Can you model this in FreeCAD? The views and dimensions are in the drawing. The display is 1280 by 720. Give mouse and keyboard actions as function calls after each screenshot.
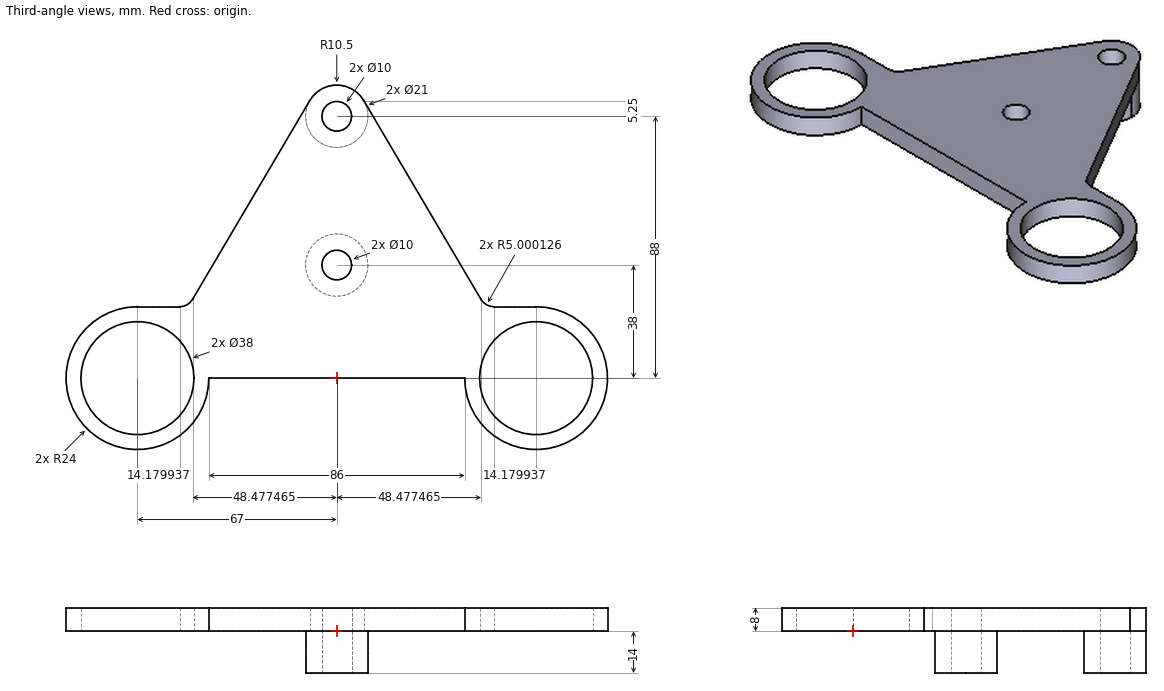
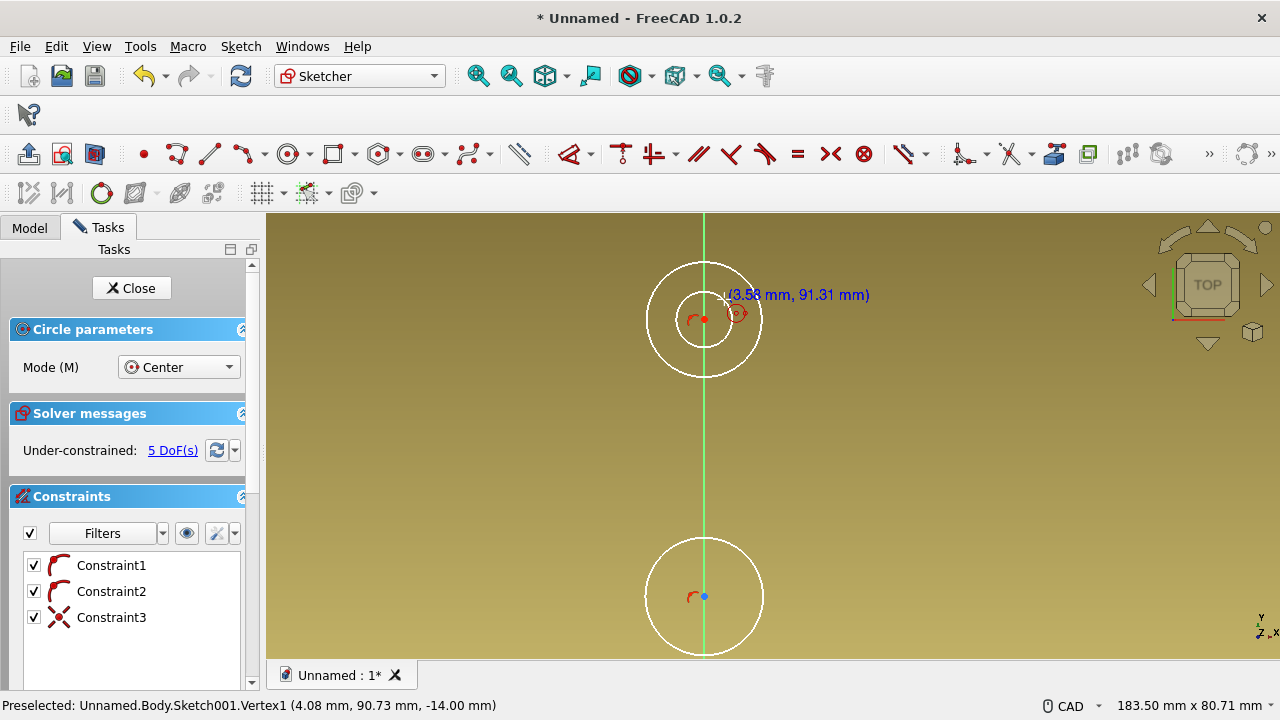
click(704, 597)
click(724, 575)
key(Escape)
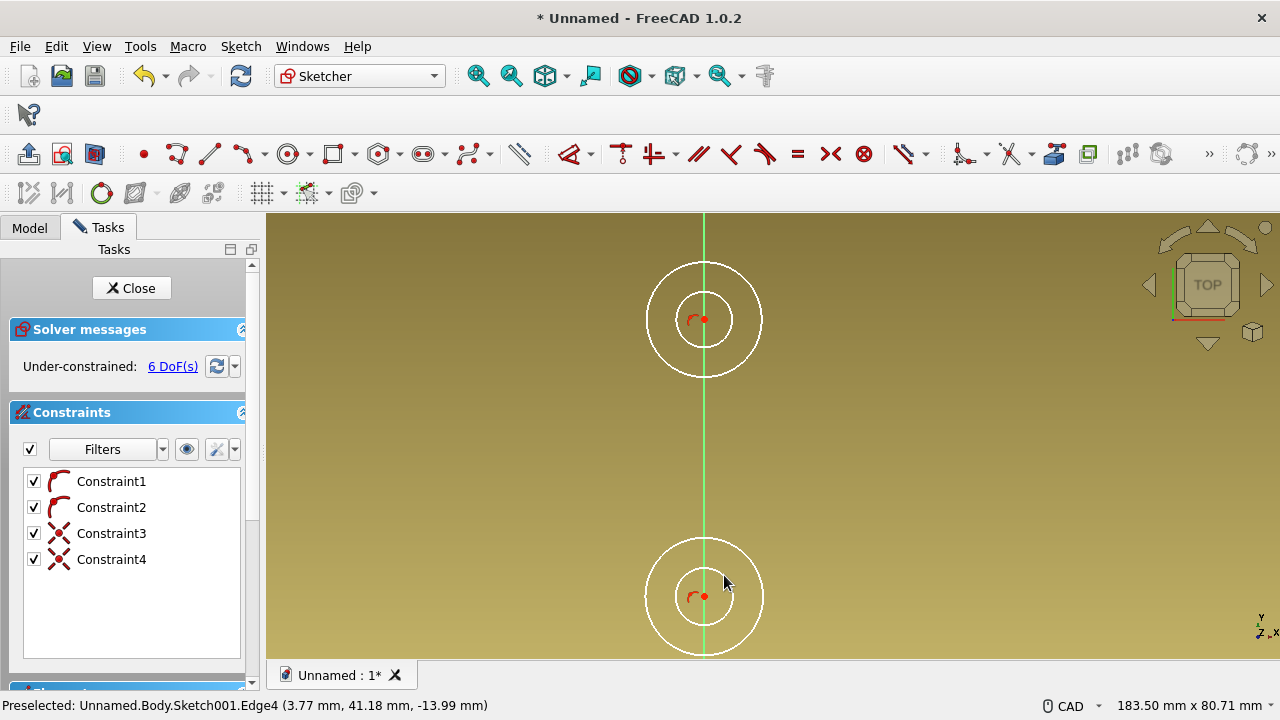
click(745, 279)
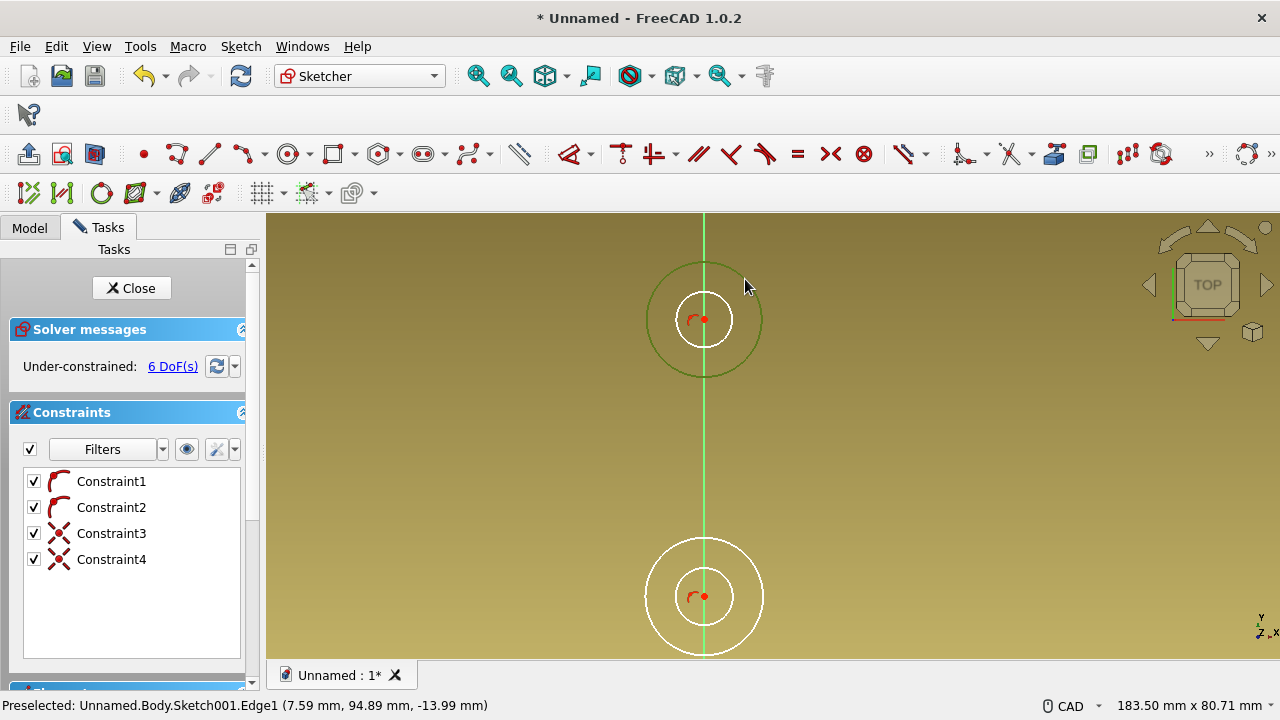
click(746, 555)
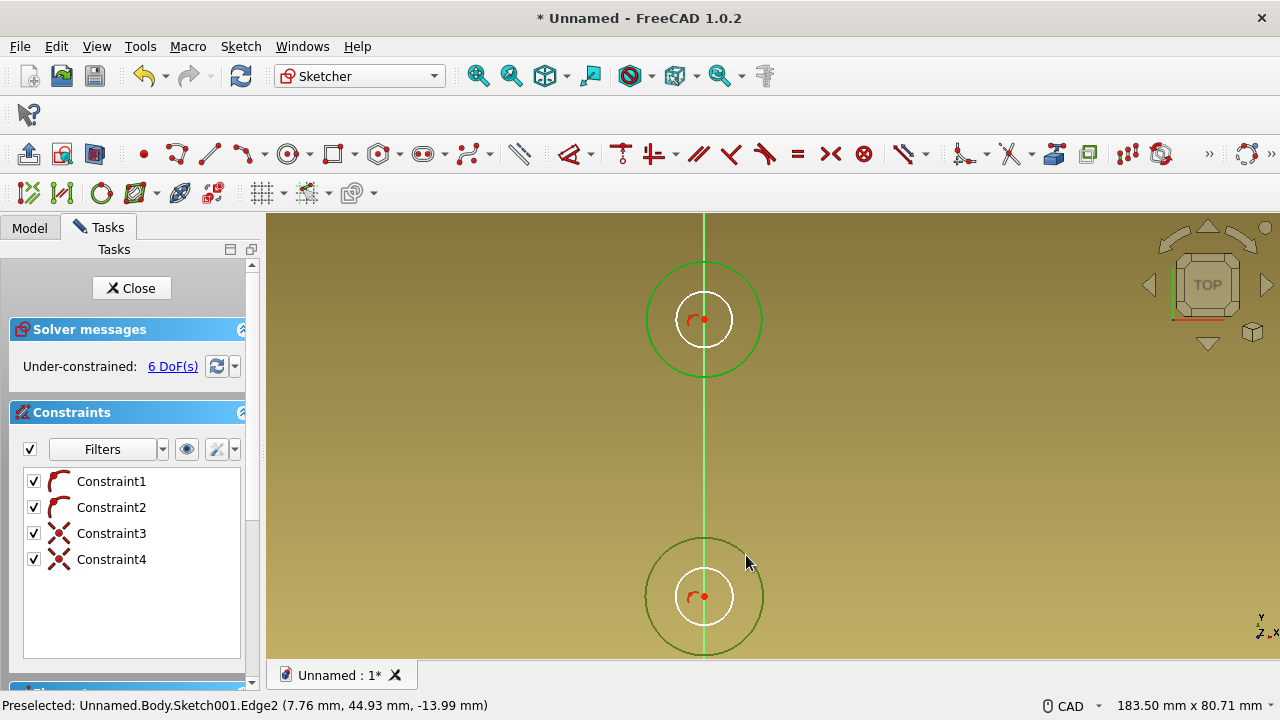
click(798, 154)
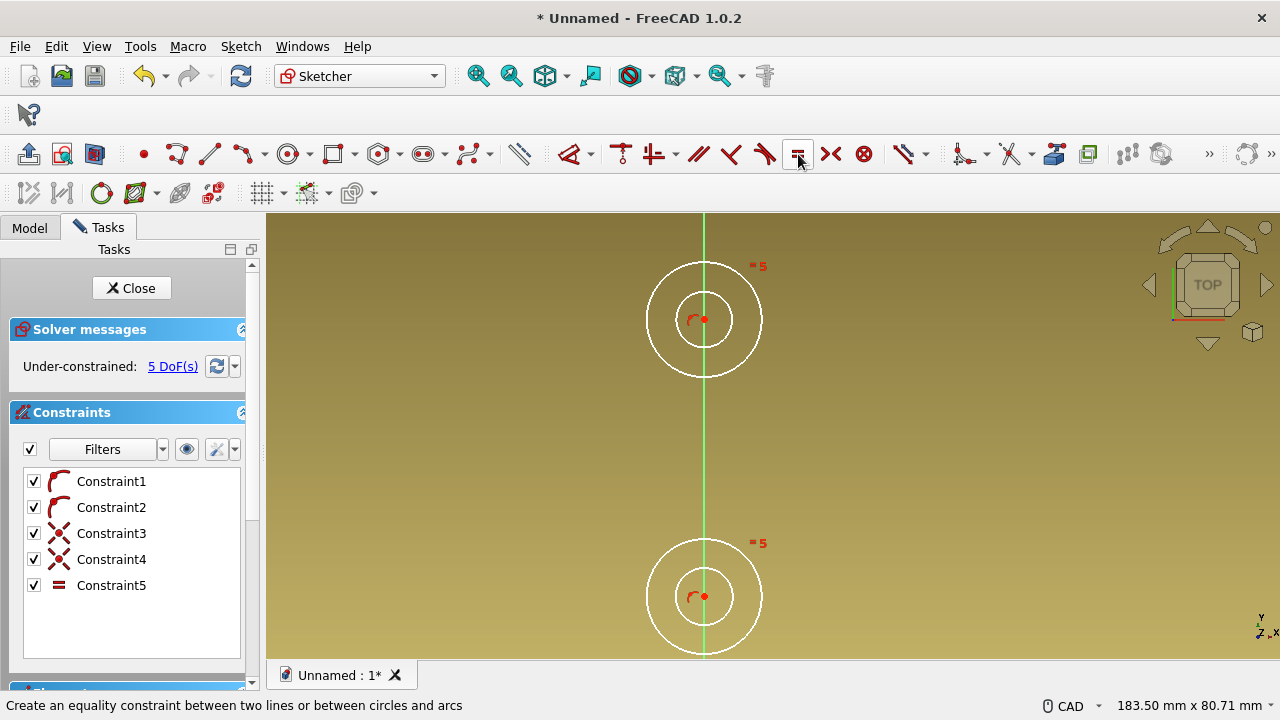
click(724, 300)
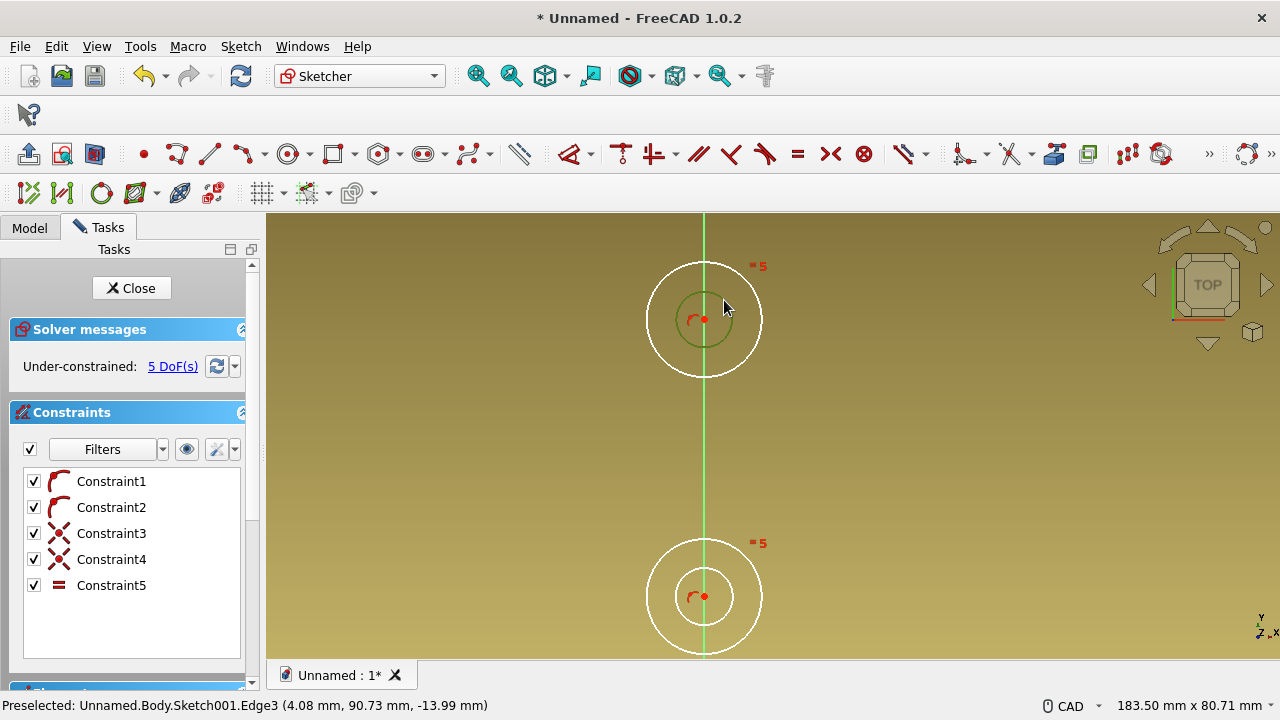
click(724, 576)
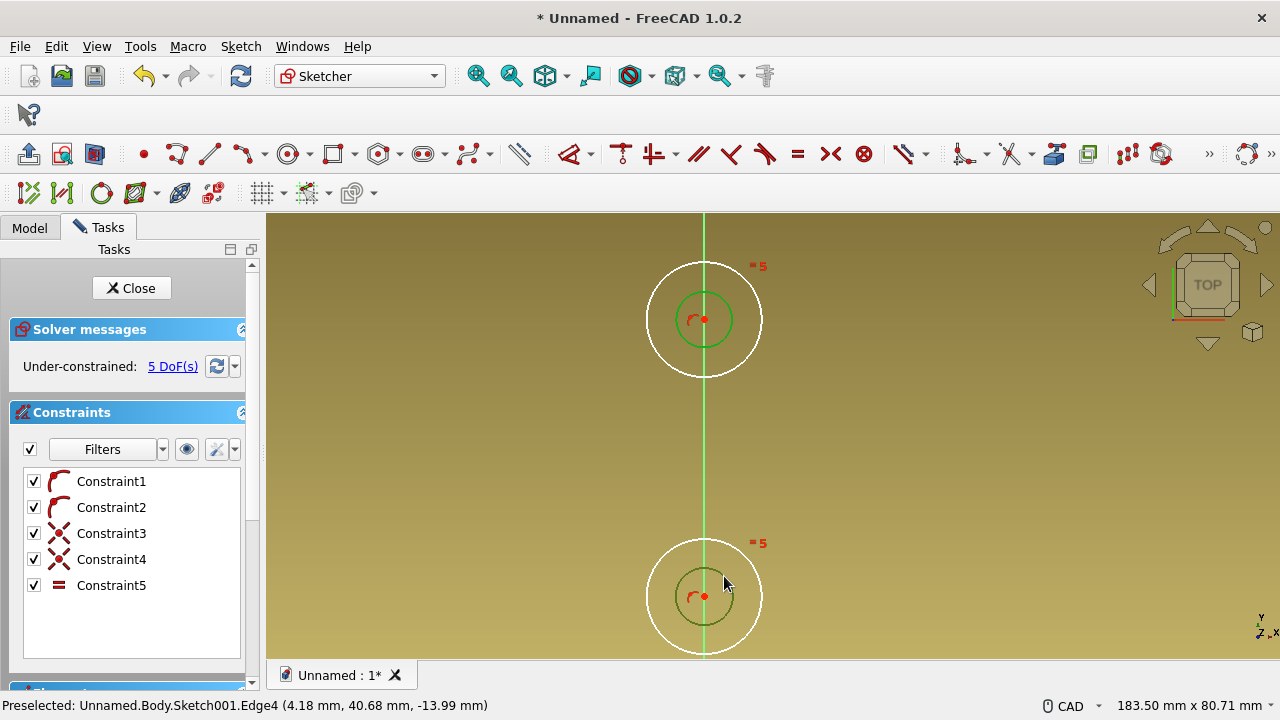
key(e)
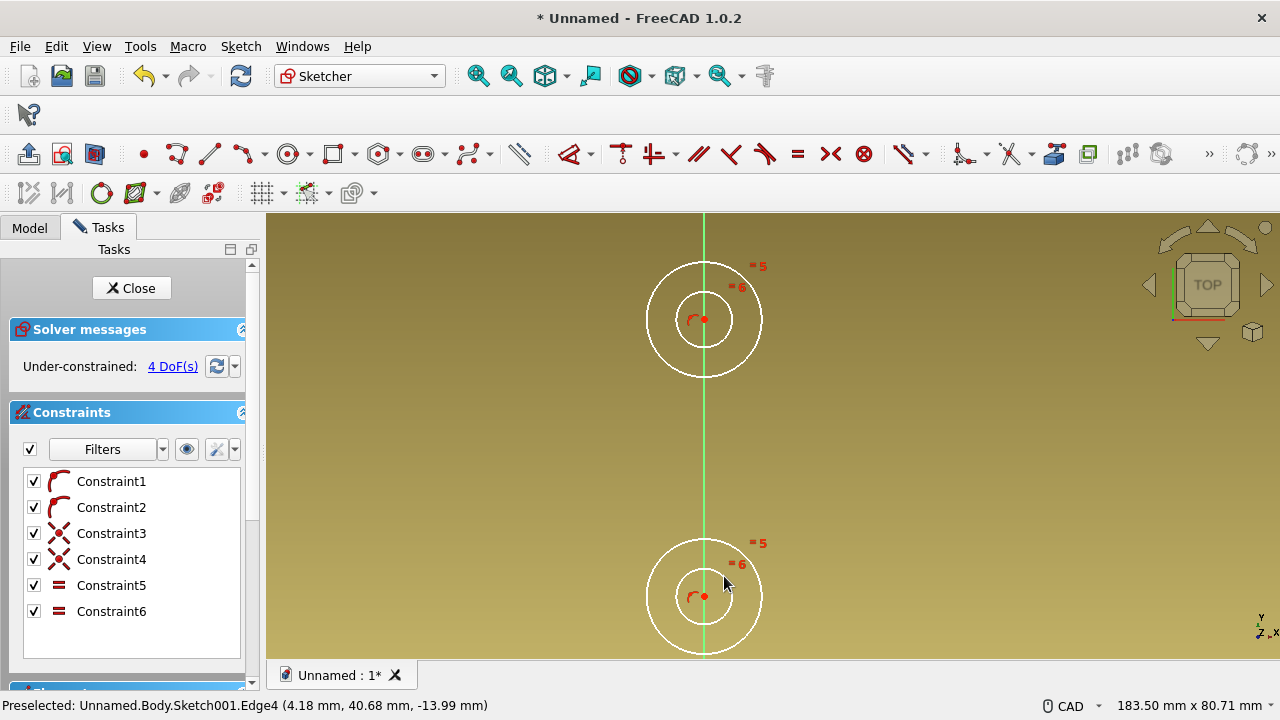
key(d)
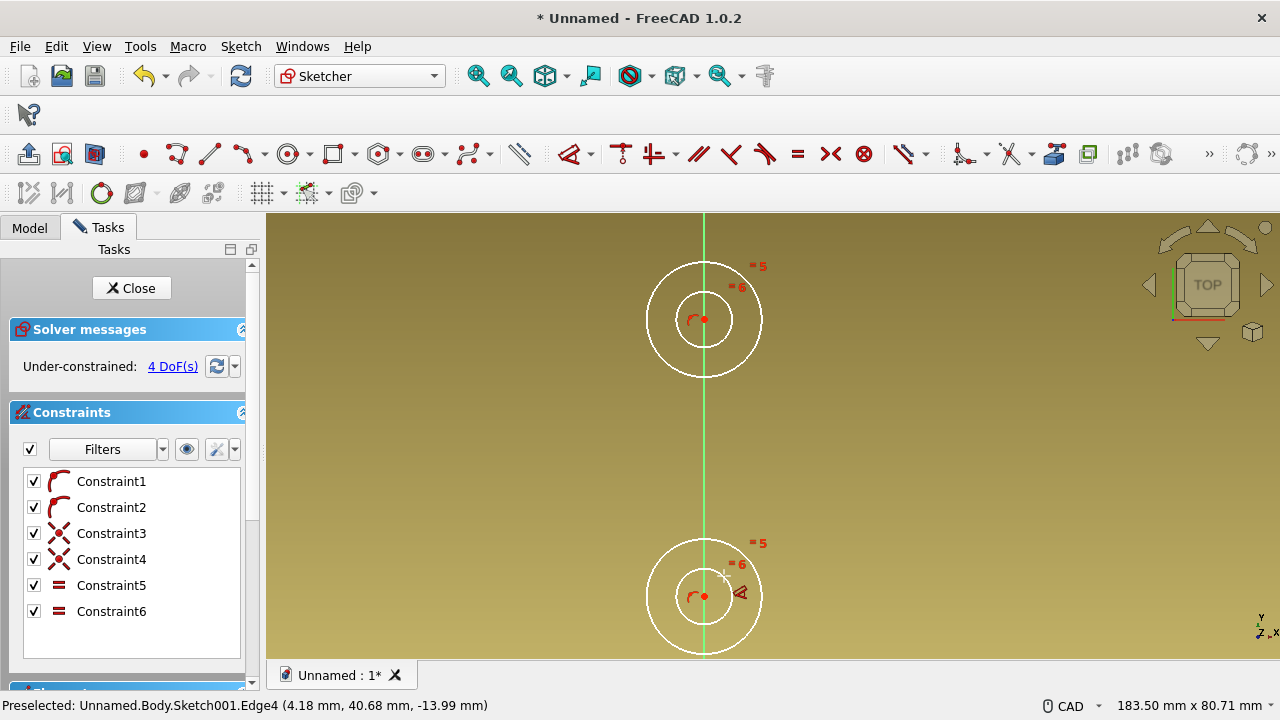
click(745, 279)
click(768, 256)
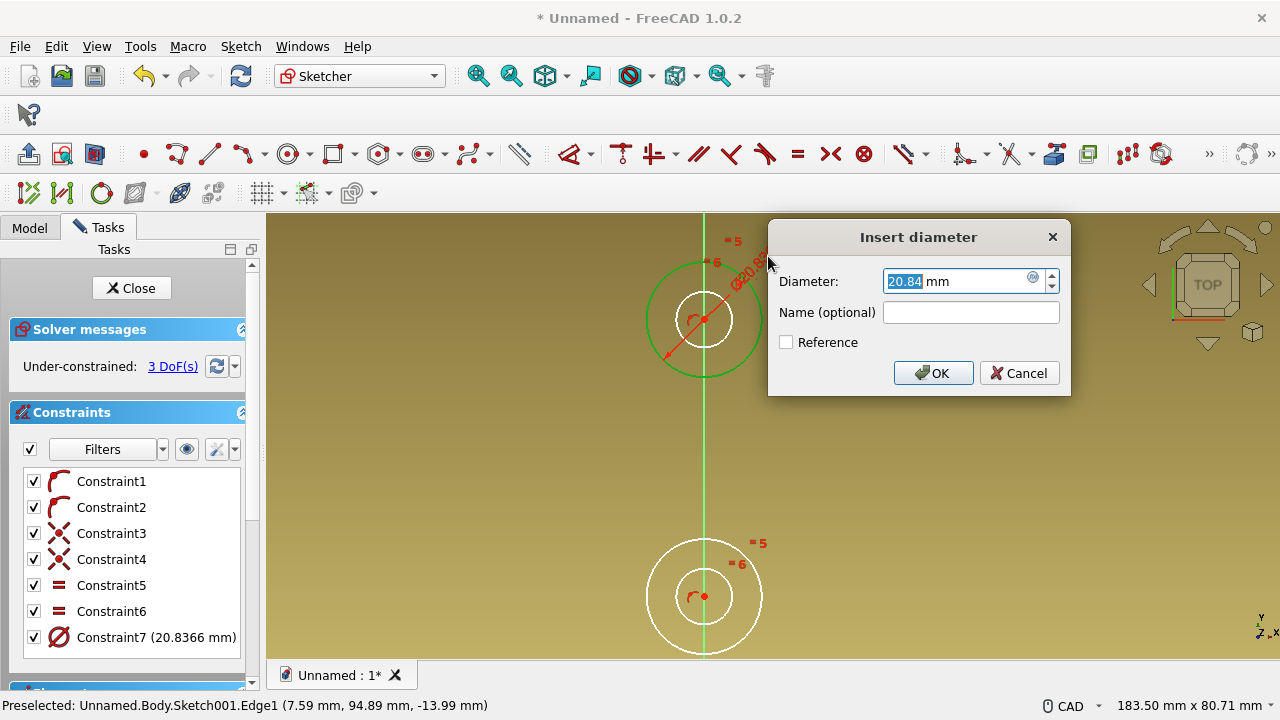
text(21)
key(Return)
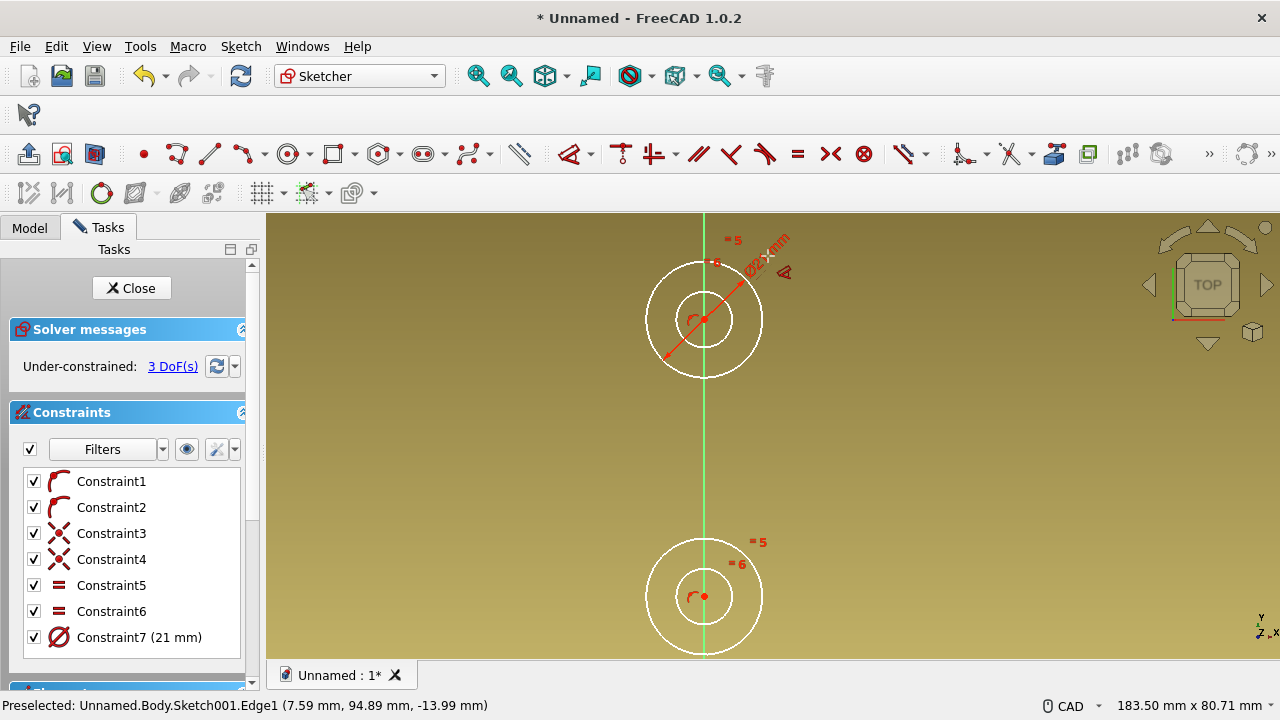
click(724, 300)
click(784, 297)